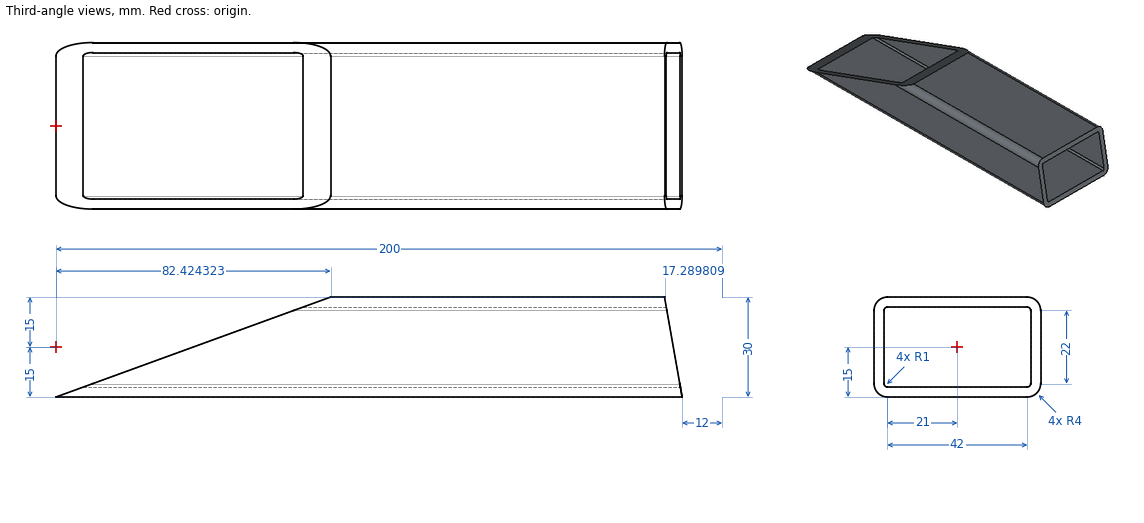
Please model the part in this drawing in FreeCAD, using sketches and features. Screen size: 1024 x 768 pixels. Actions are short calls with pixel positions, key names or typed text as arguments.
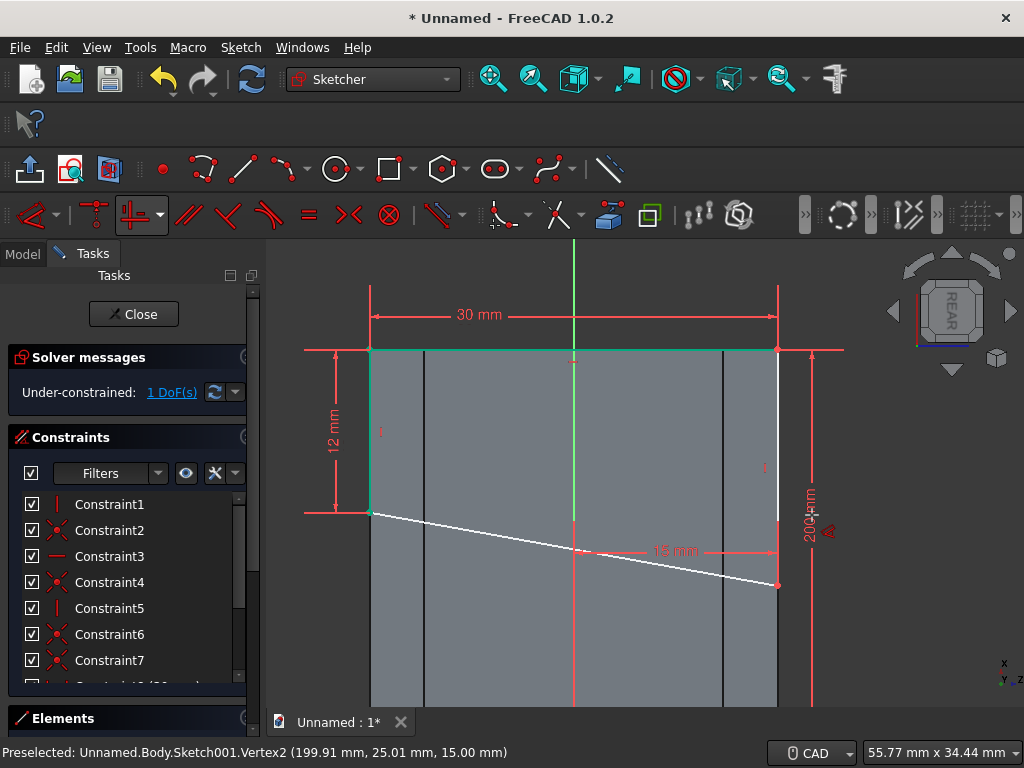
click(778, 515)
click(812, 468)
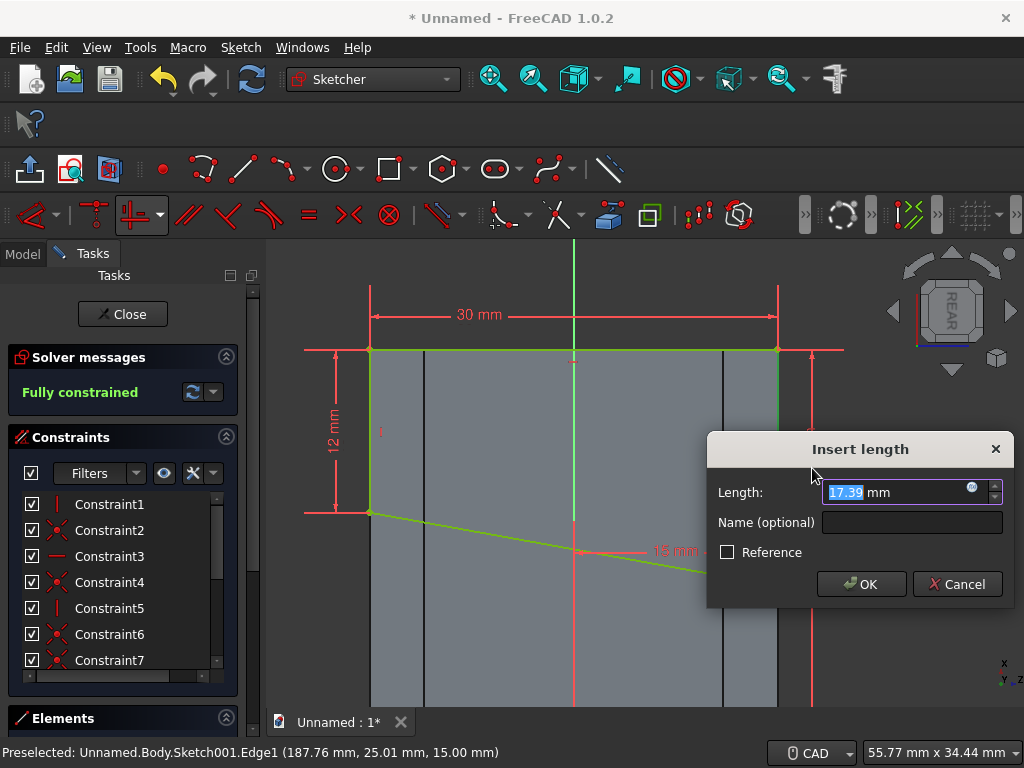
text(17.289809)
key(Return)
key(Escape)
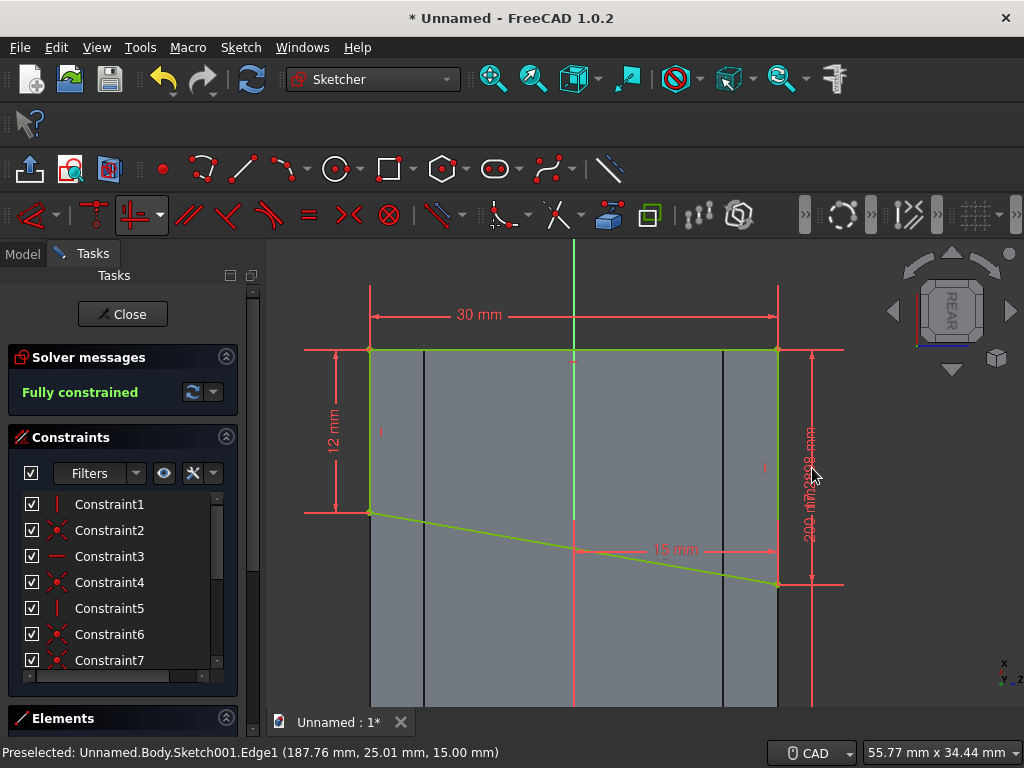
click(123, 314)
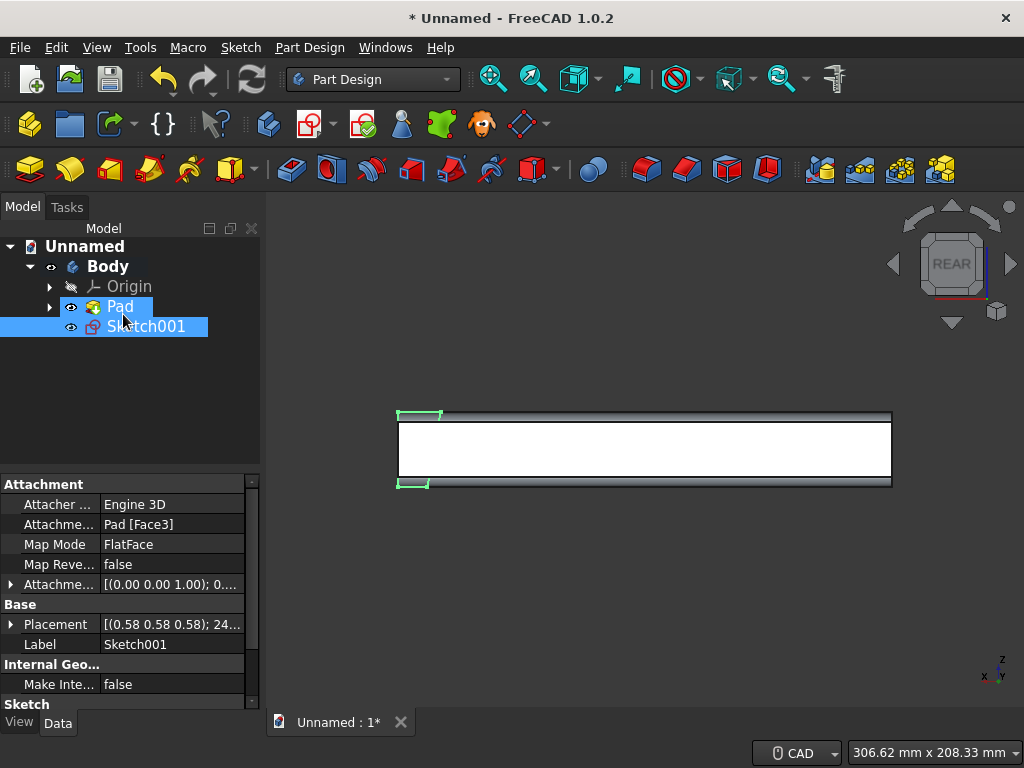
click(292, 170)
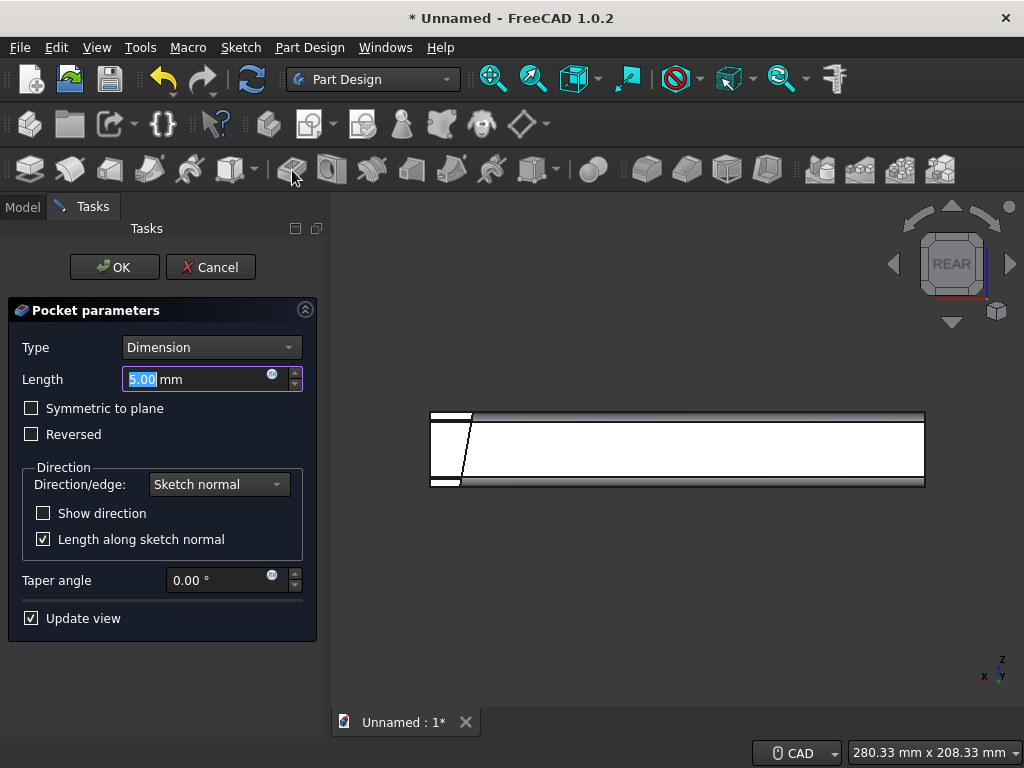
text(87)
key(Tab)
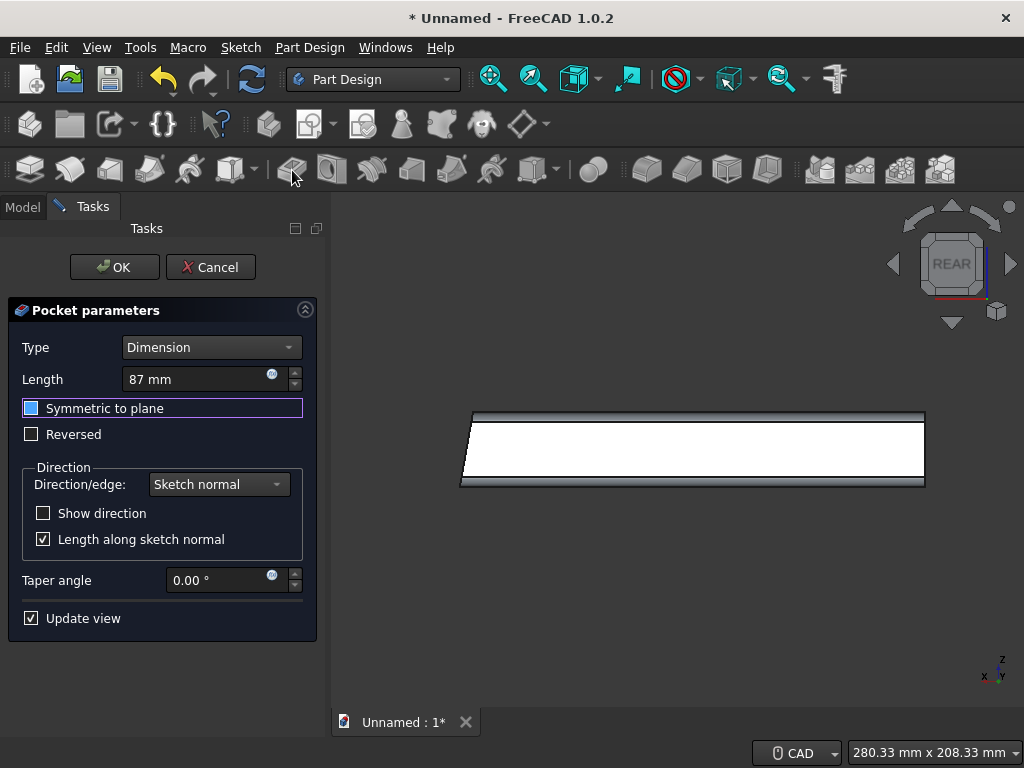
click(115, 267)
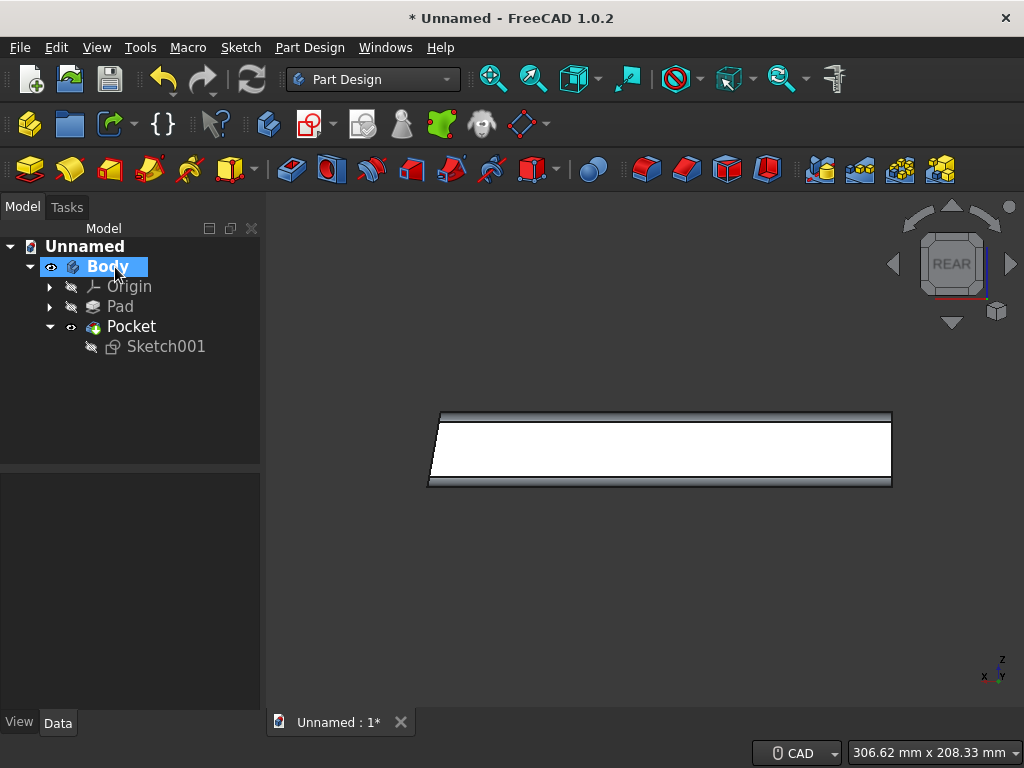
click(661, 449)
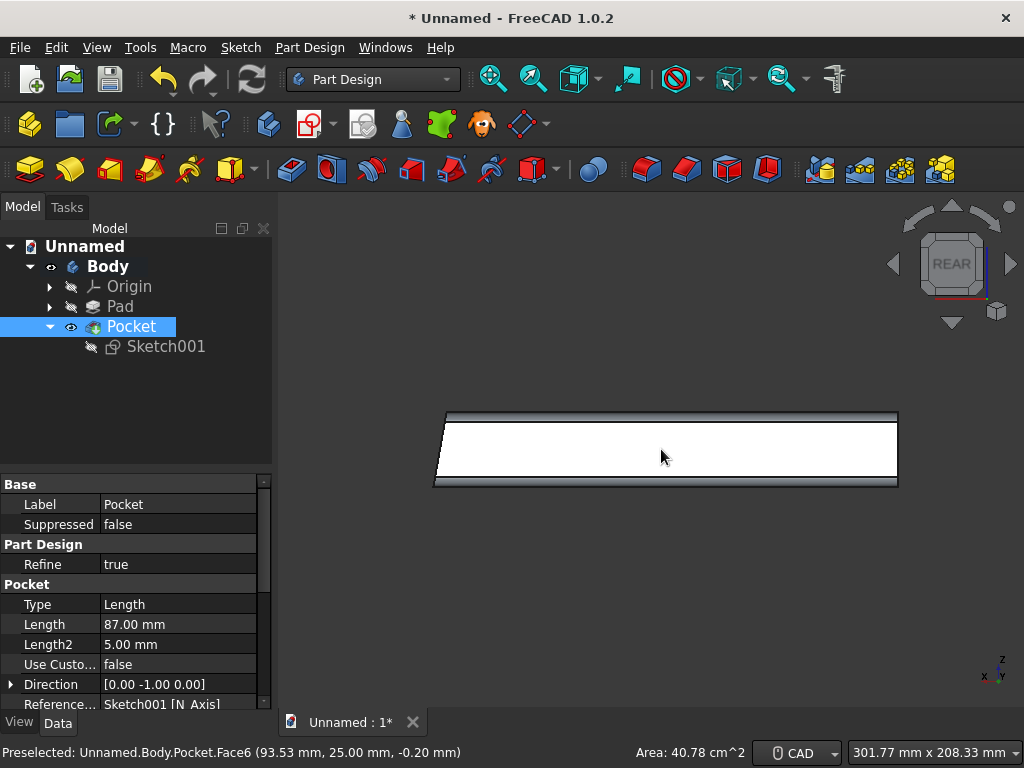
click(310, 124)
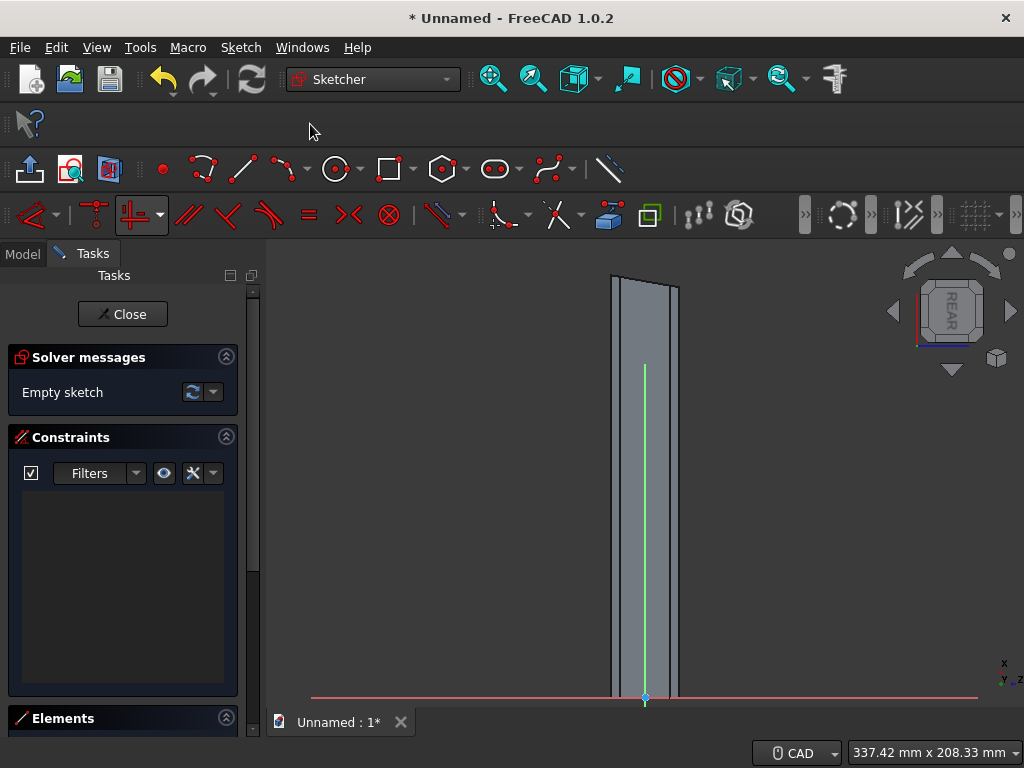
scroll(294, 267, down, 1)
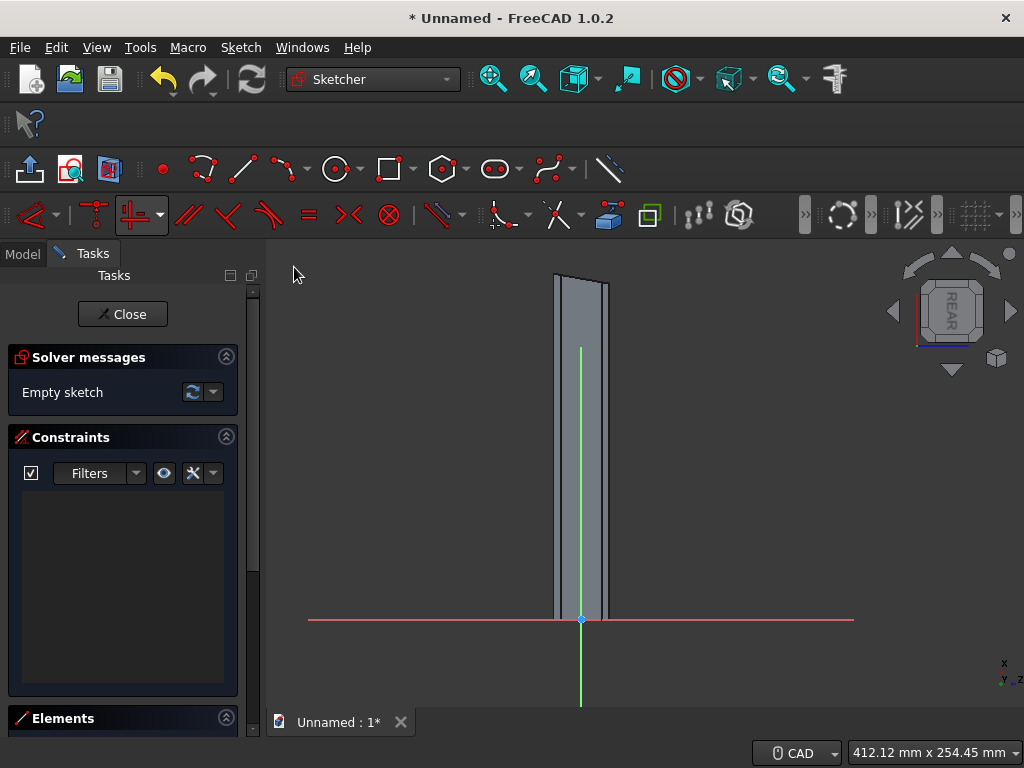
scroll(587, 630, up, 3)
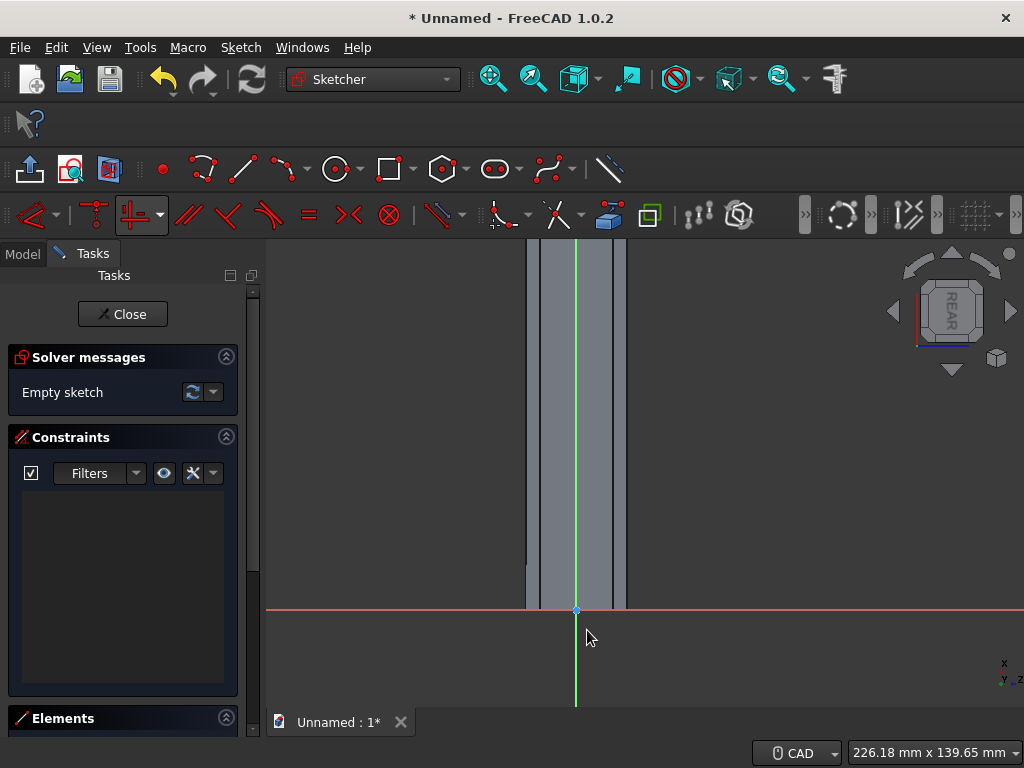
click(204, 170)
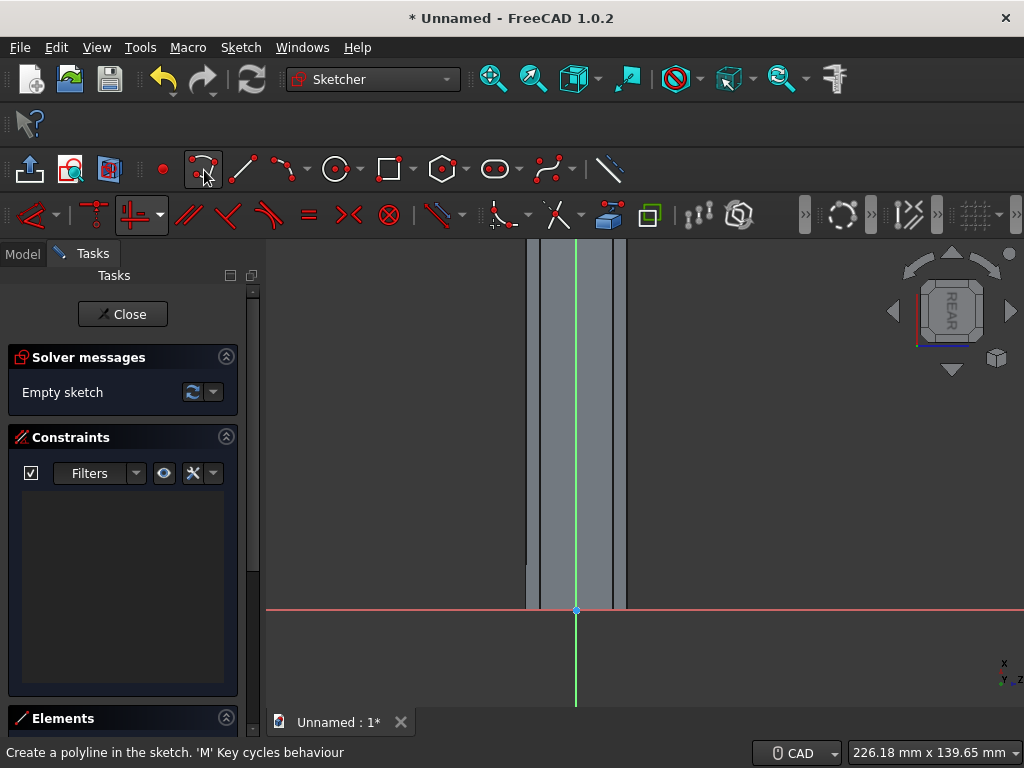
click(526, 610)
click(627, 601)
click(627, 334)
click(526, 610)
key(Escape)
key(Escape)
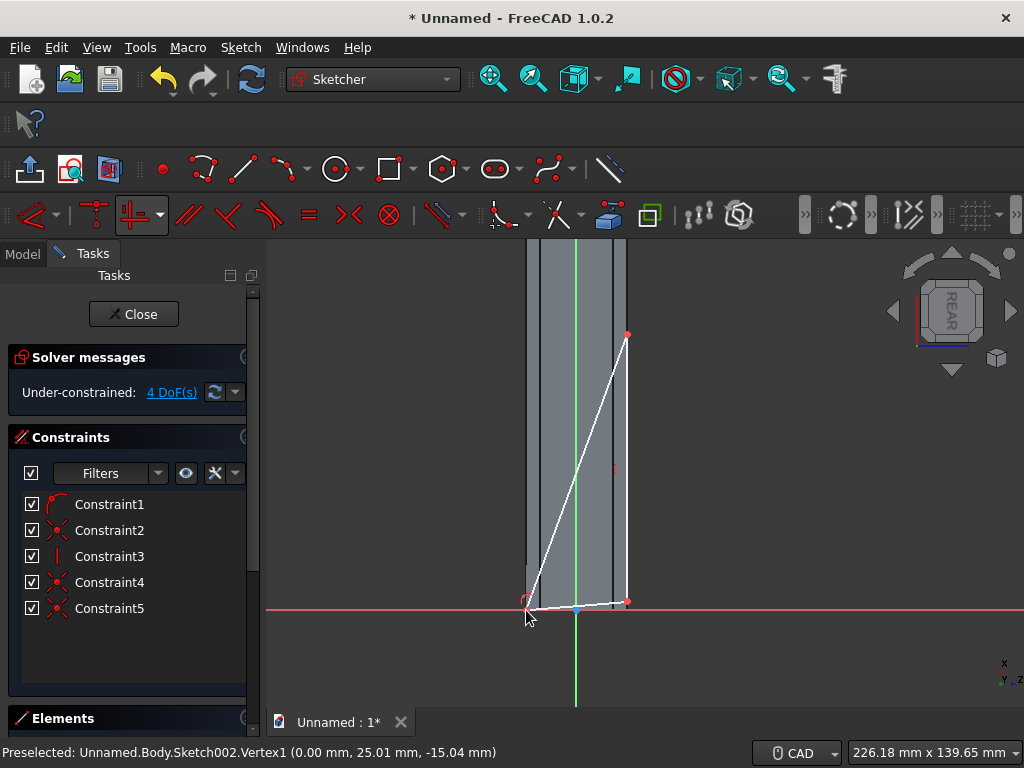
click(556, 608)